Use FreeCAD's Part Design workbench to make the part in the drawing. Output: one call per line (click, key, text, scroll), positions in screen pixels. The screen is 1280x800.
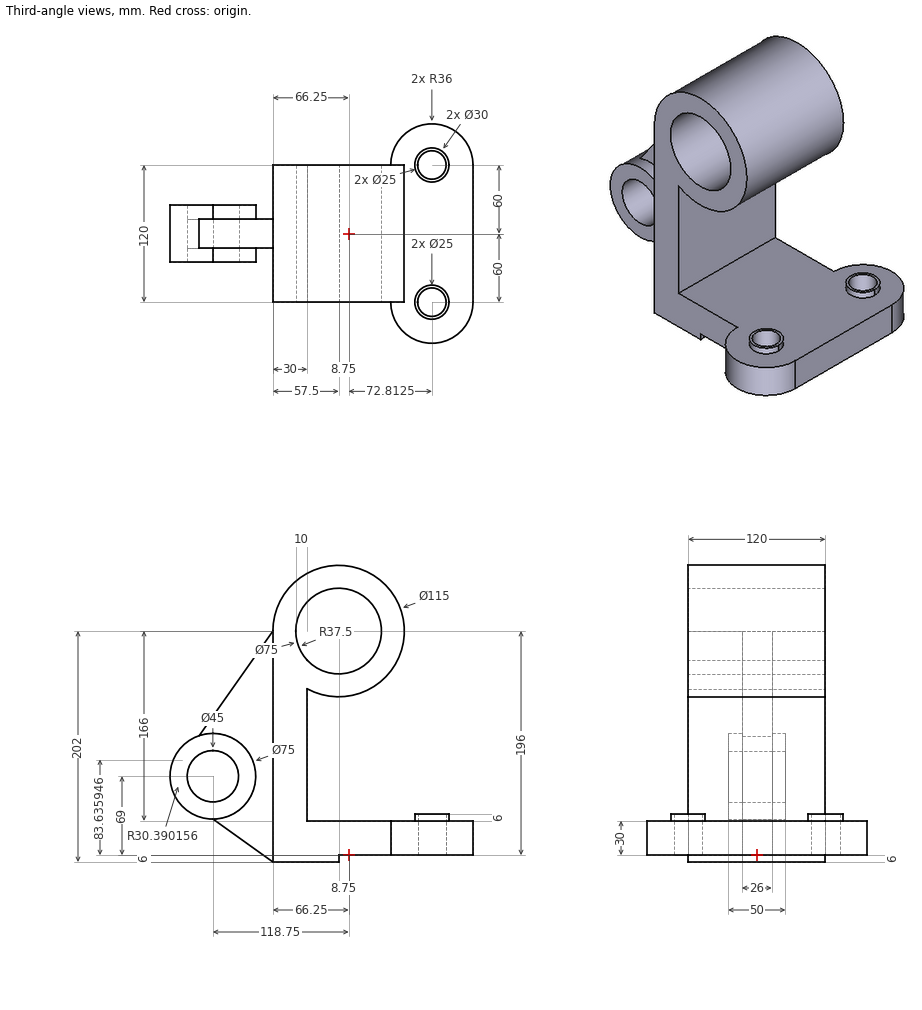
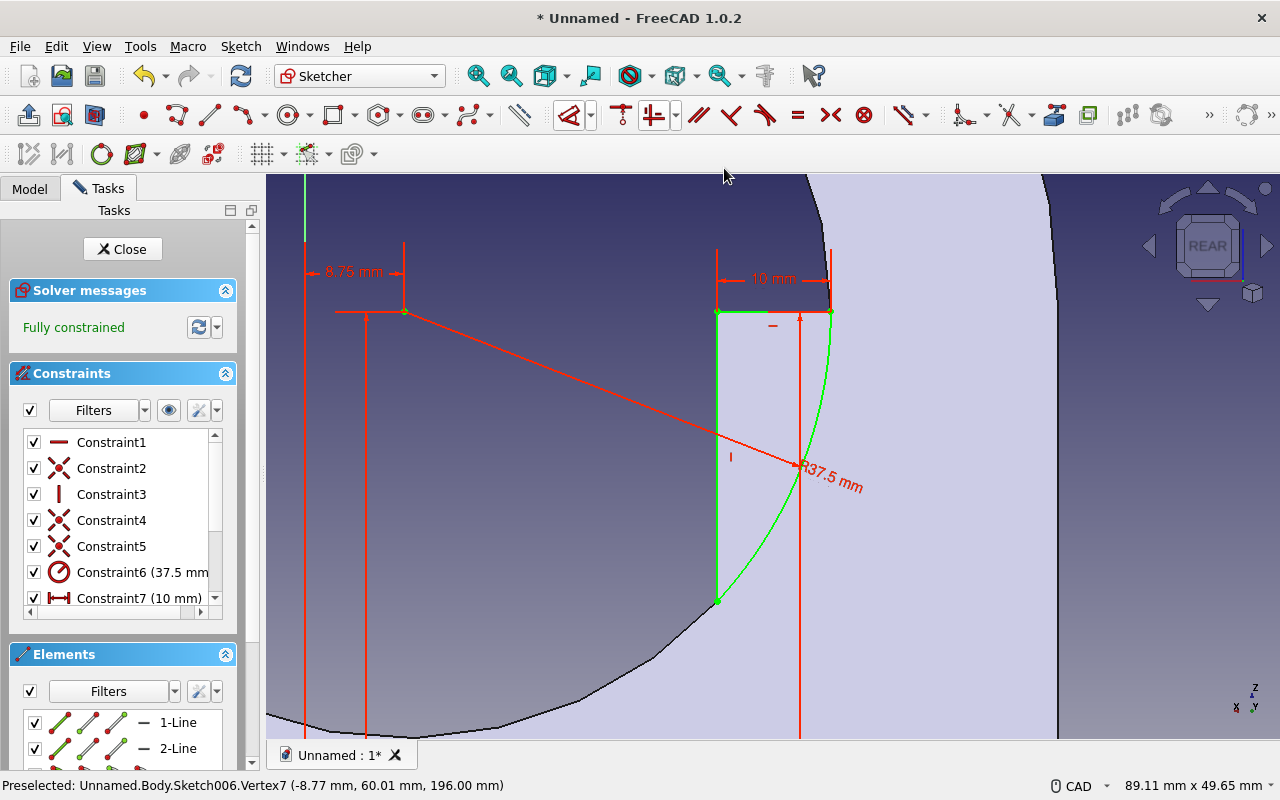
click(123, 249)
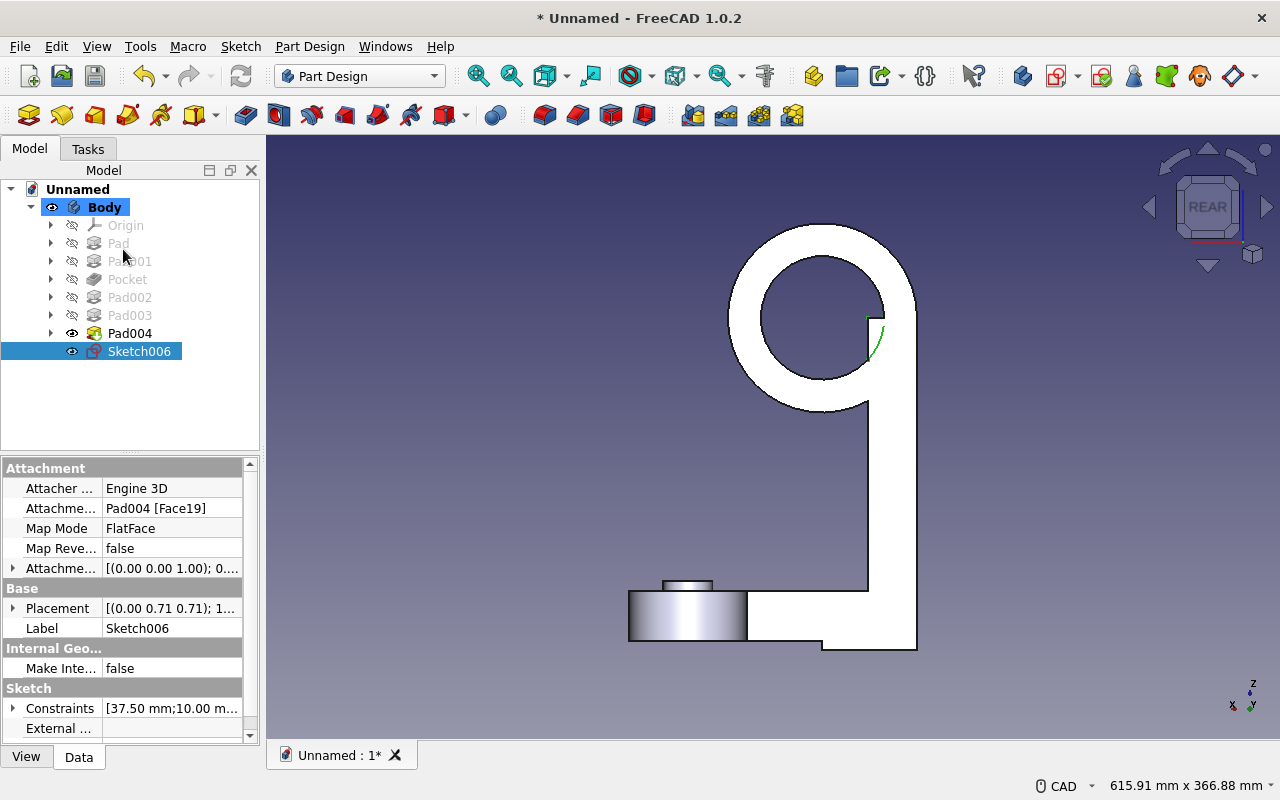
click(246, 116)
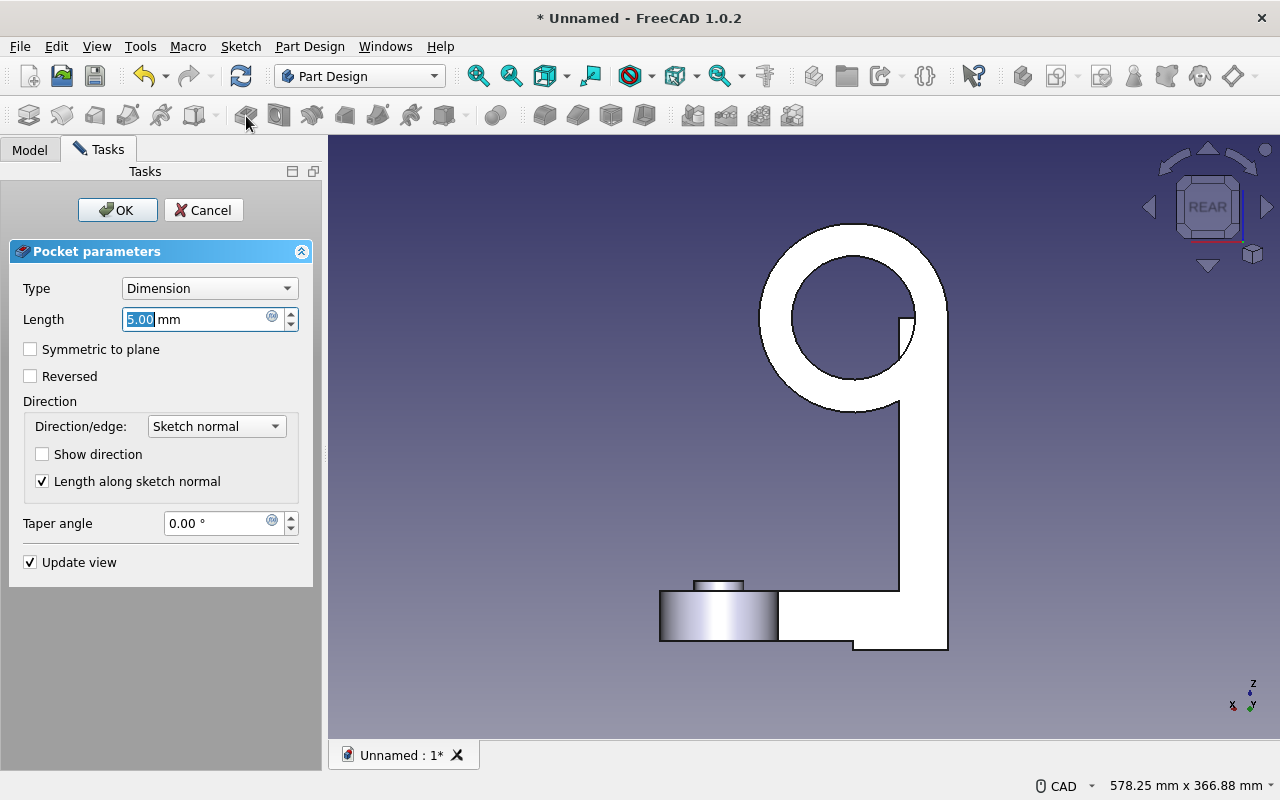
click(210, 288)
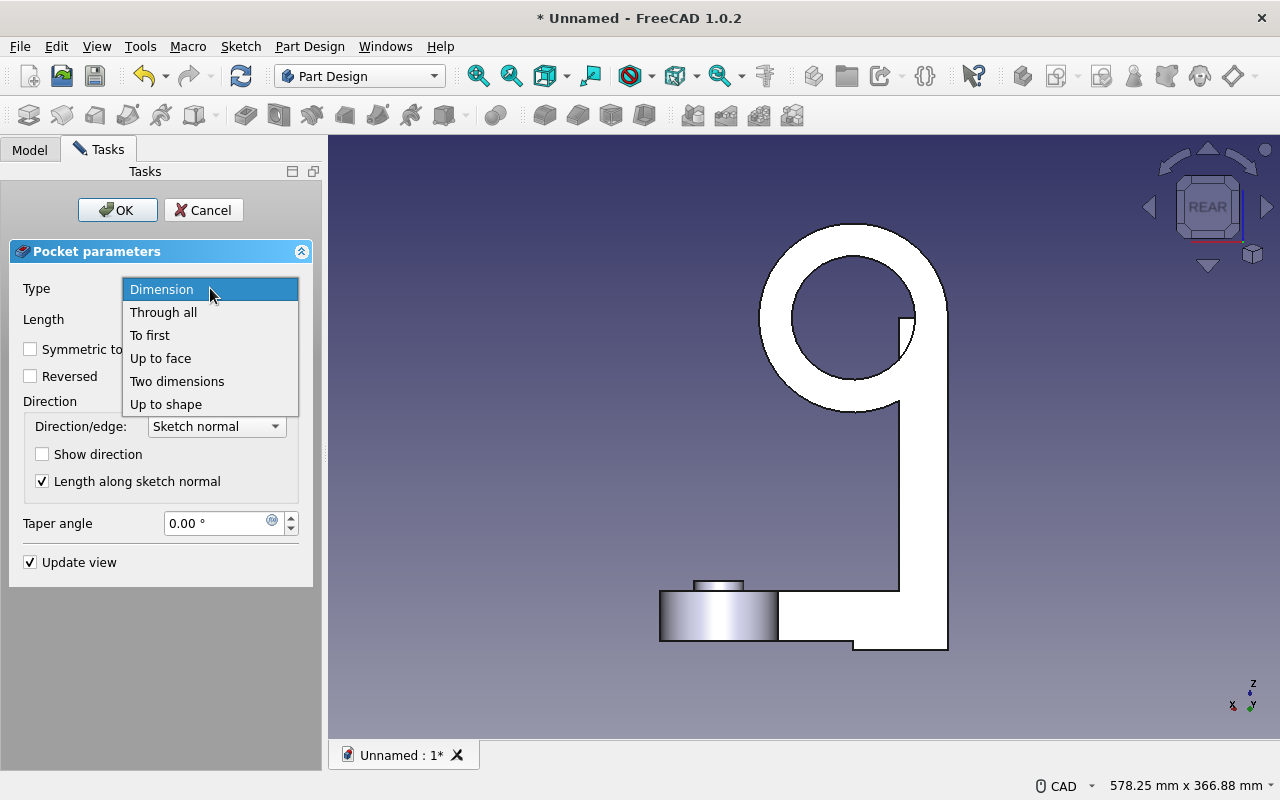
click(208, 312)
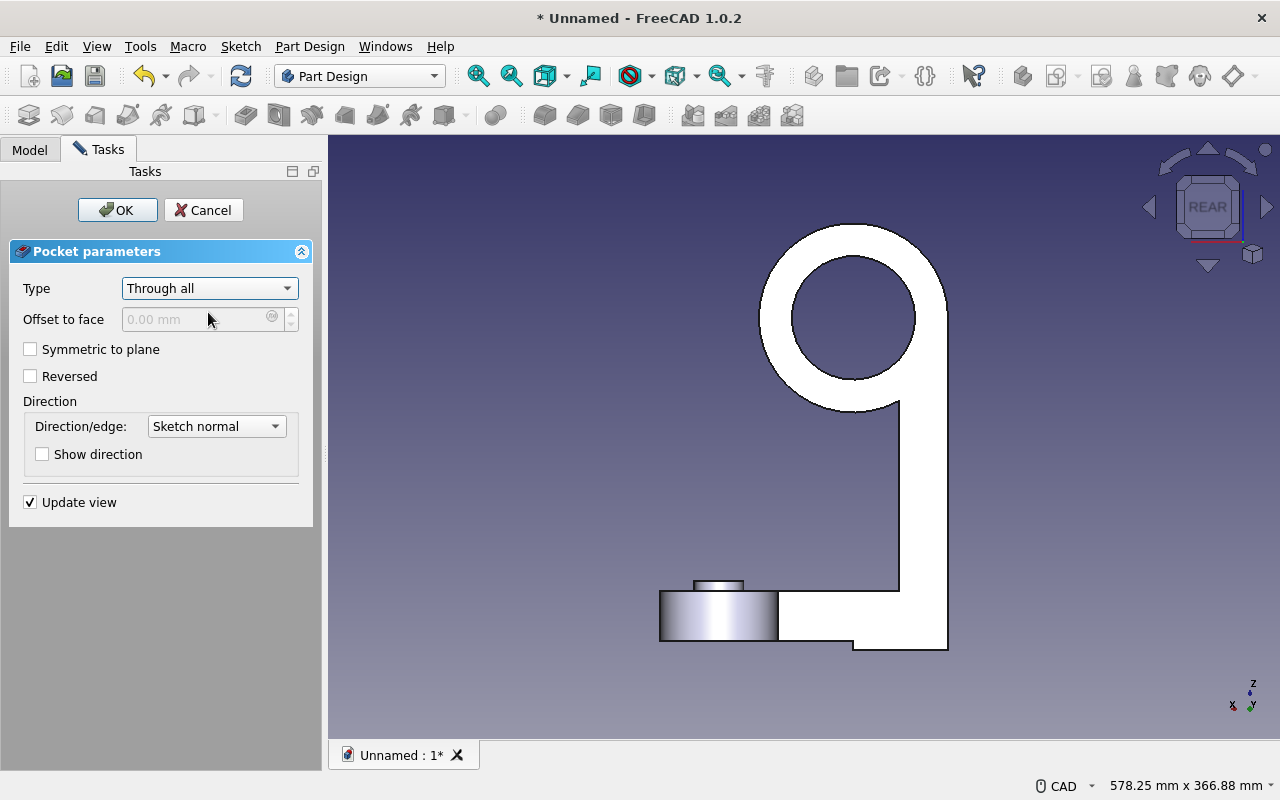
click(118, 210)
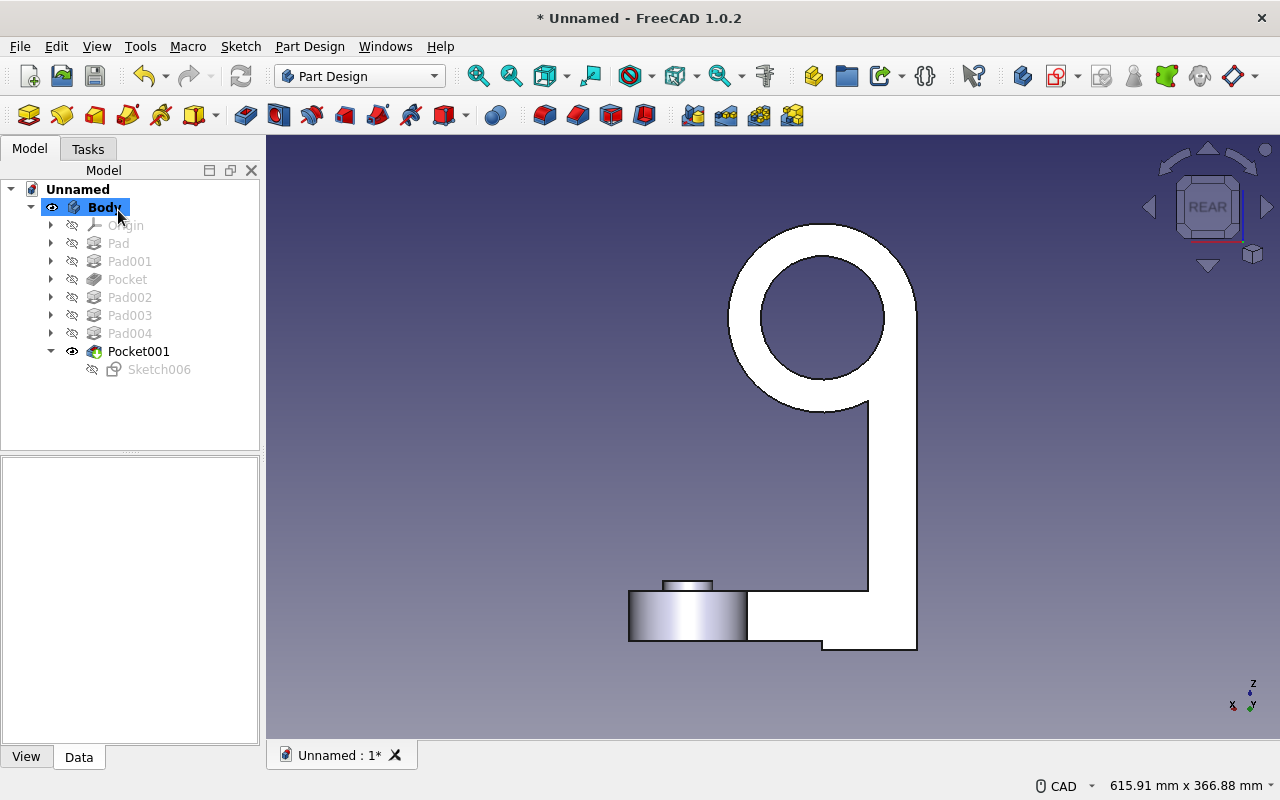
click(1056, 76)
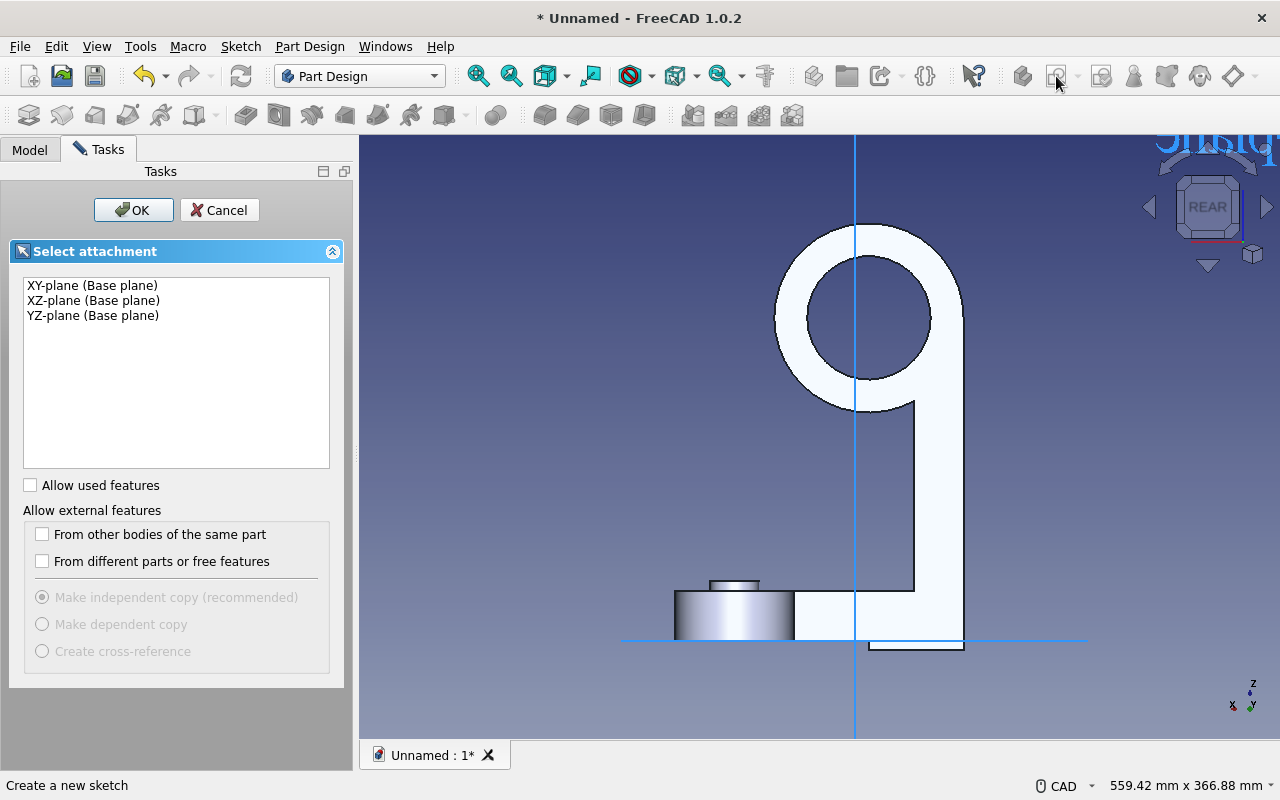
click(84, 300)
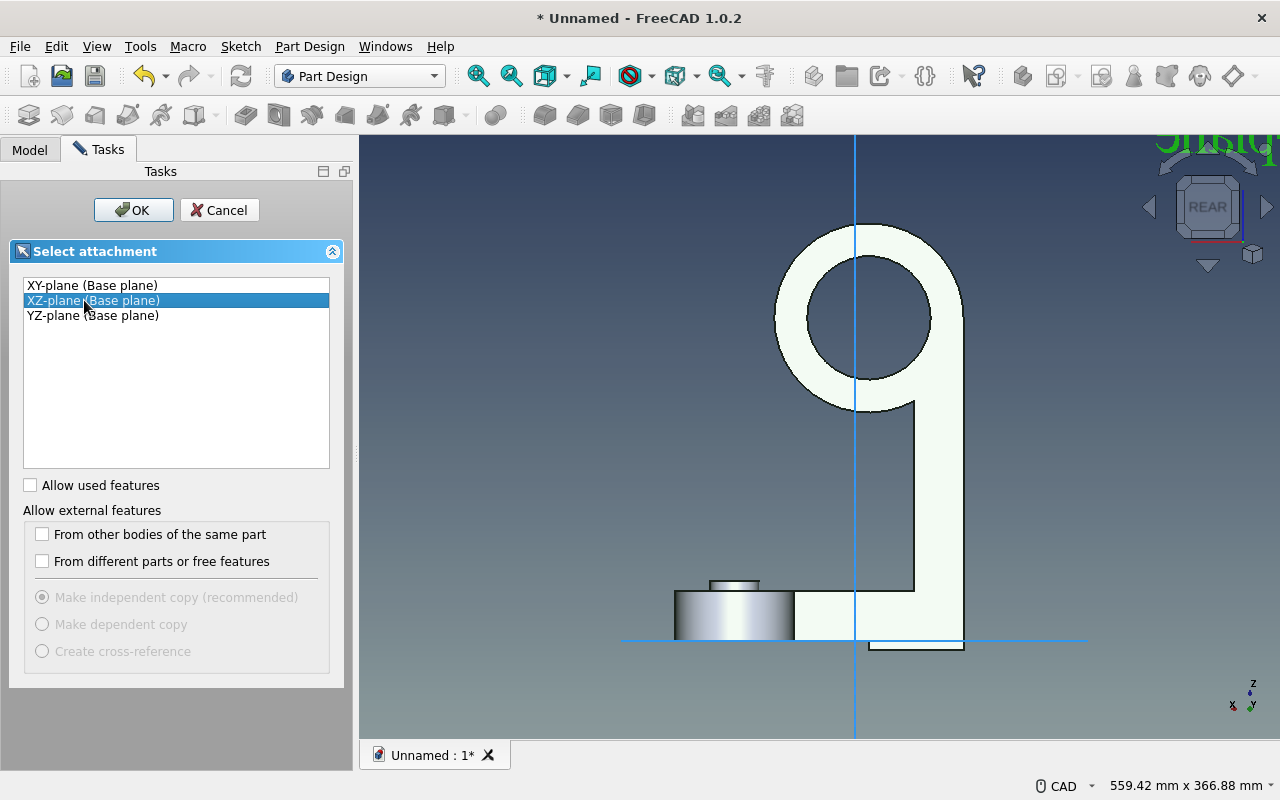
click(134, 210)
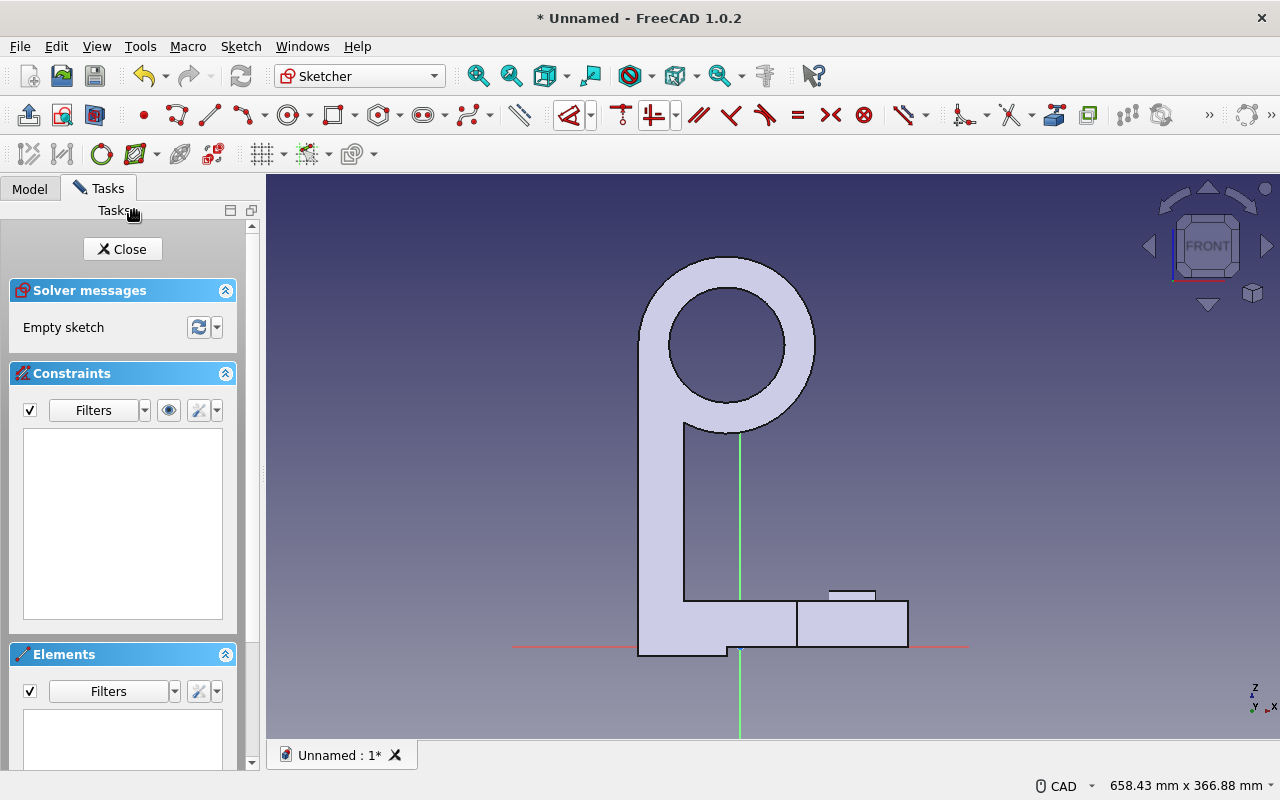
key(q)
key(s)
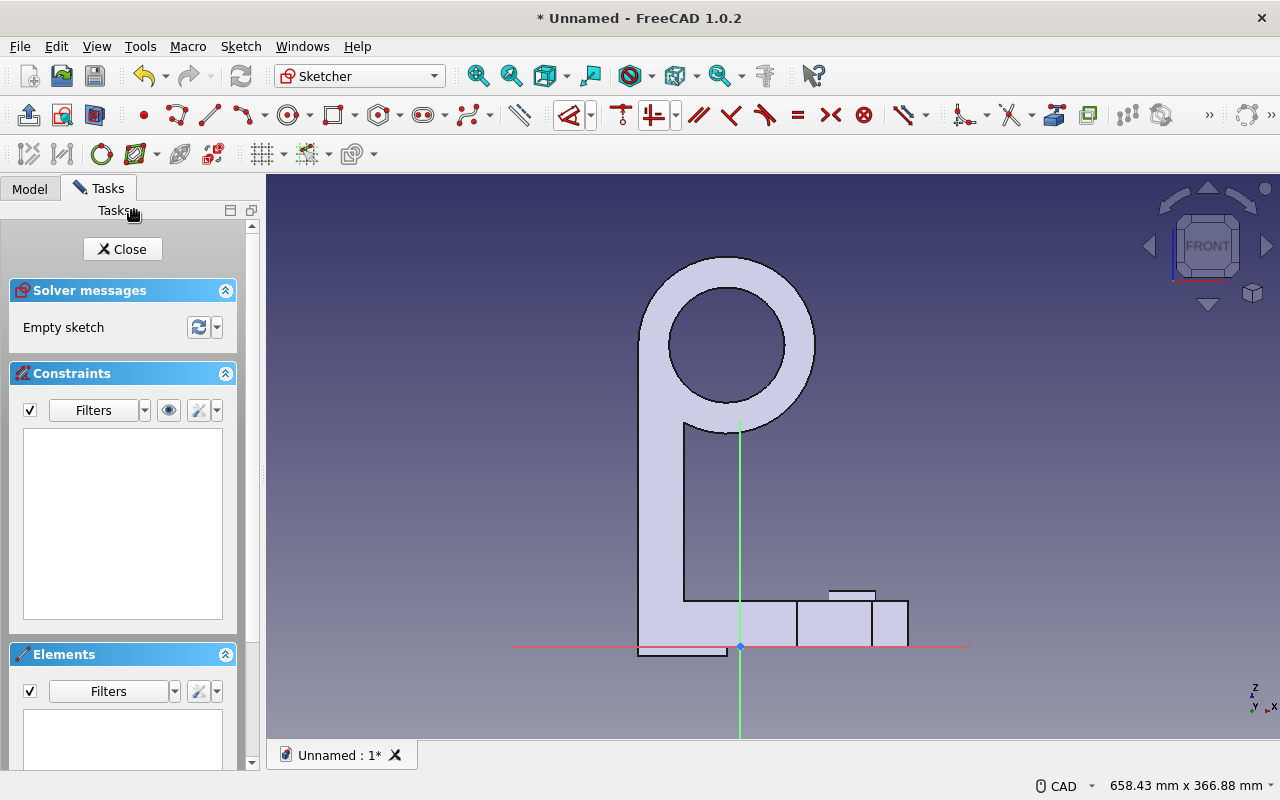
key(g)
key(m)